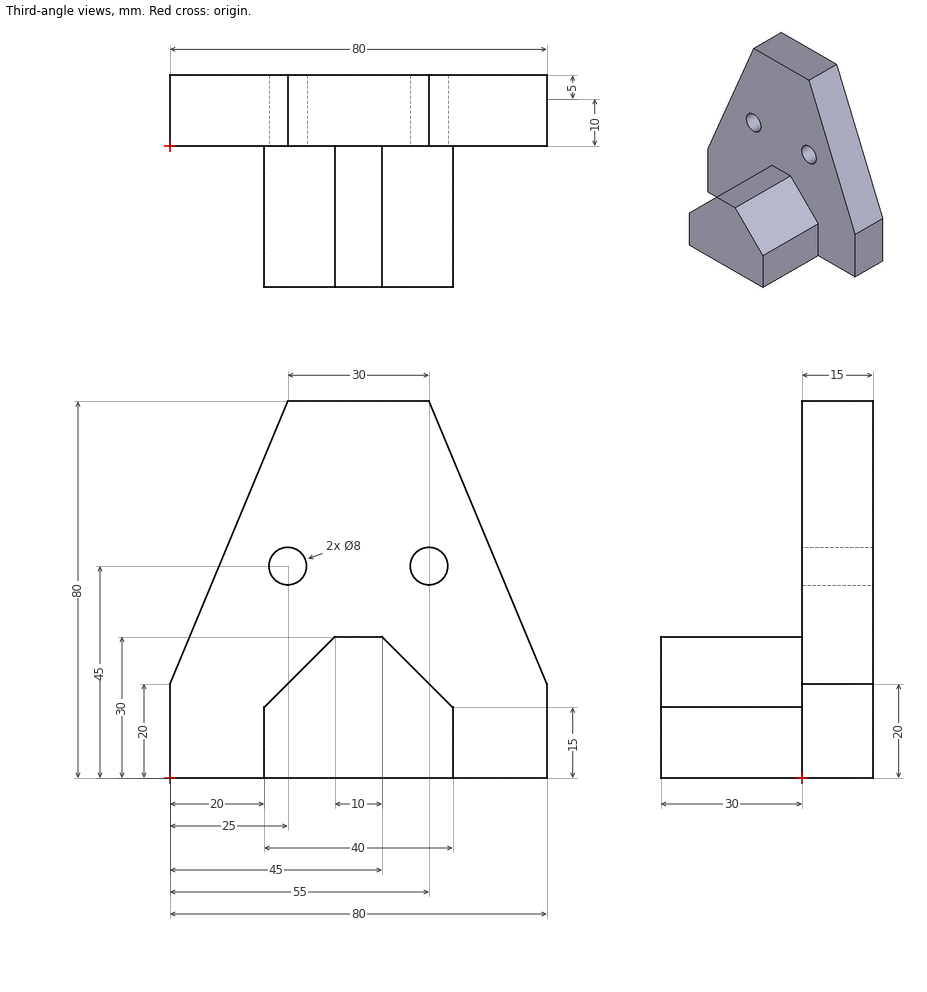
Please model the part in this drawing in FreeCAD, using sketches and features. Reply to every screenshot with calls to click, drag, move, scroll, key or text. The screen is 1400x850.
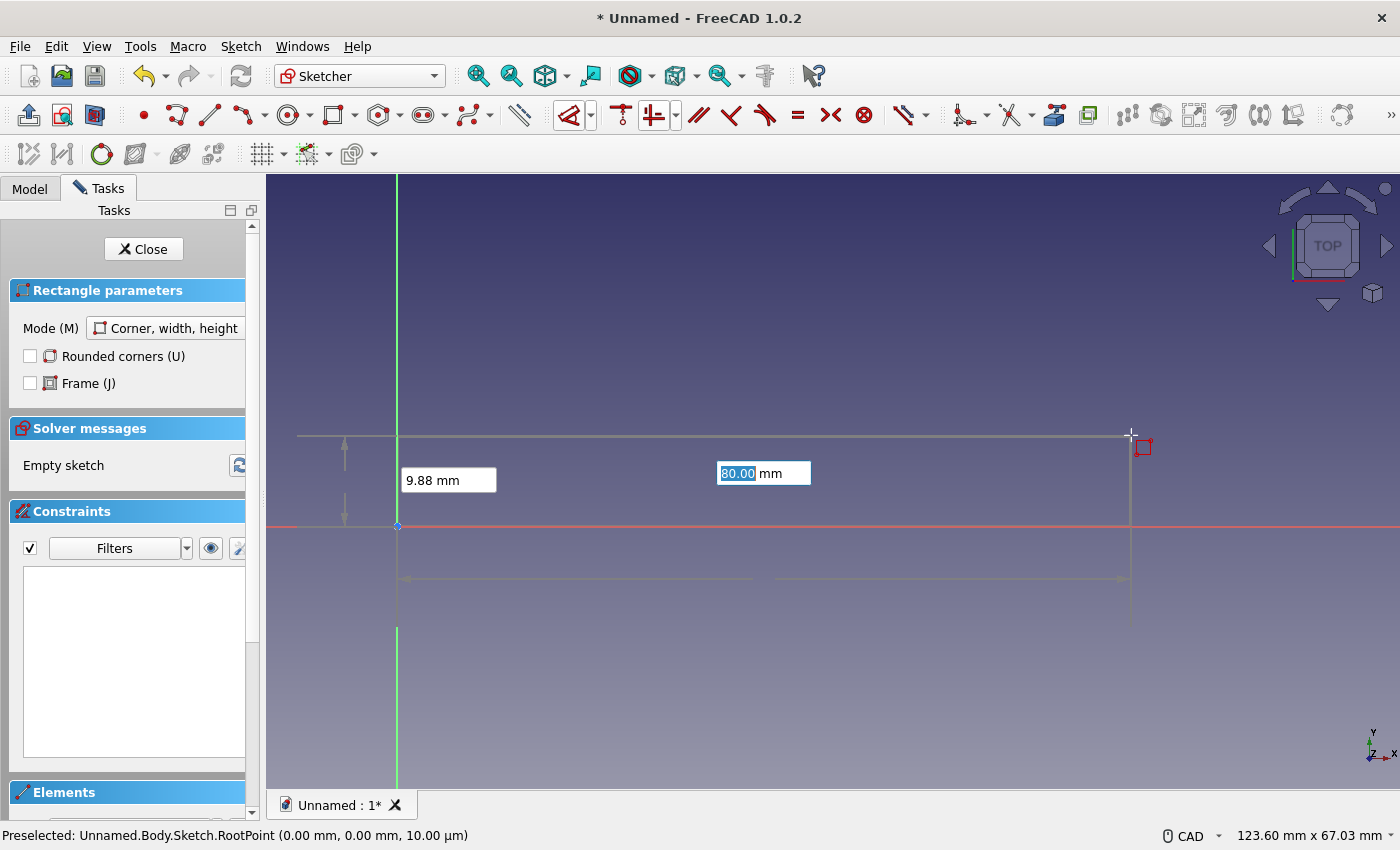
text(80)
key(Tab)
text(10)
key(Return)
key(Escape)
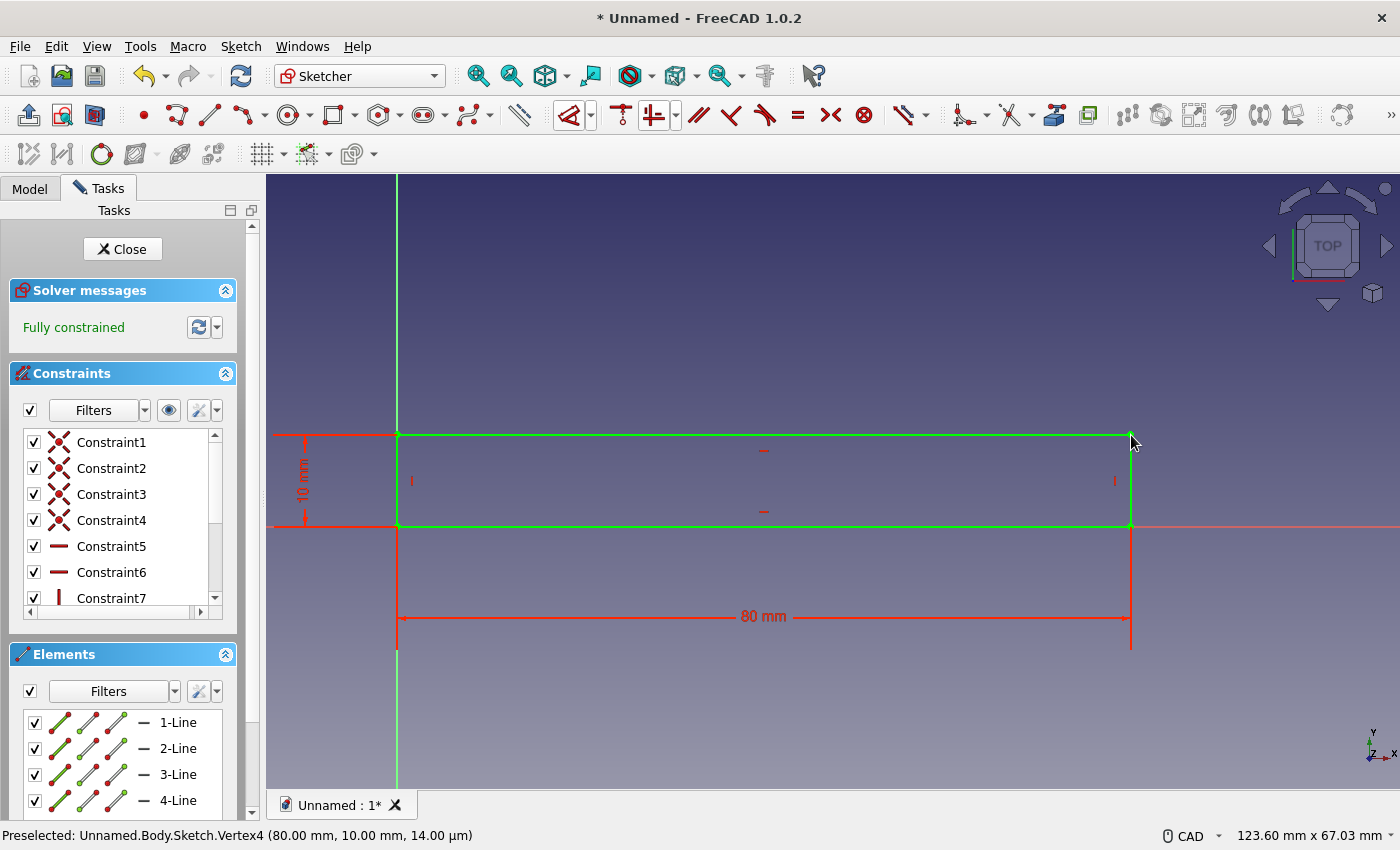
click(123, 249)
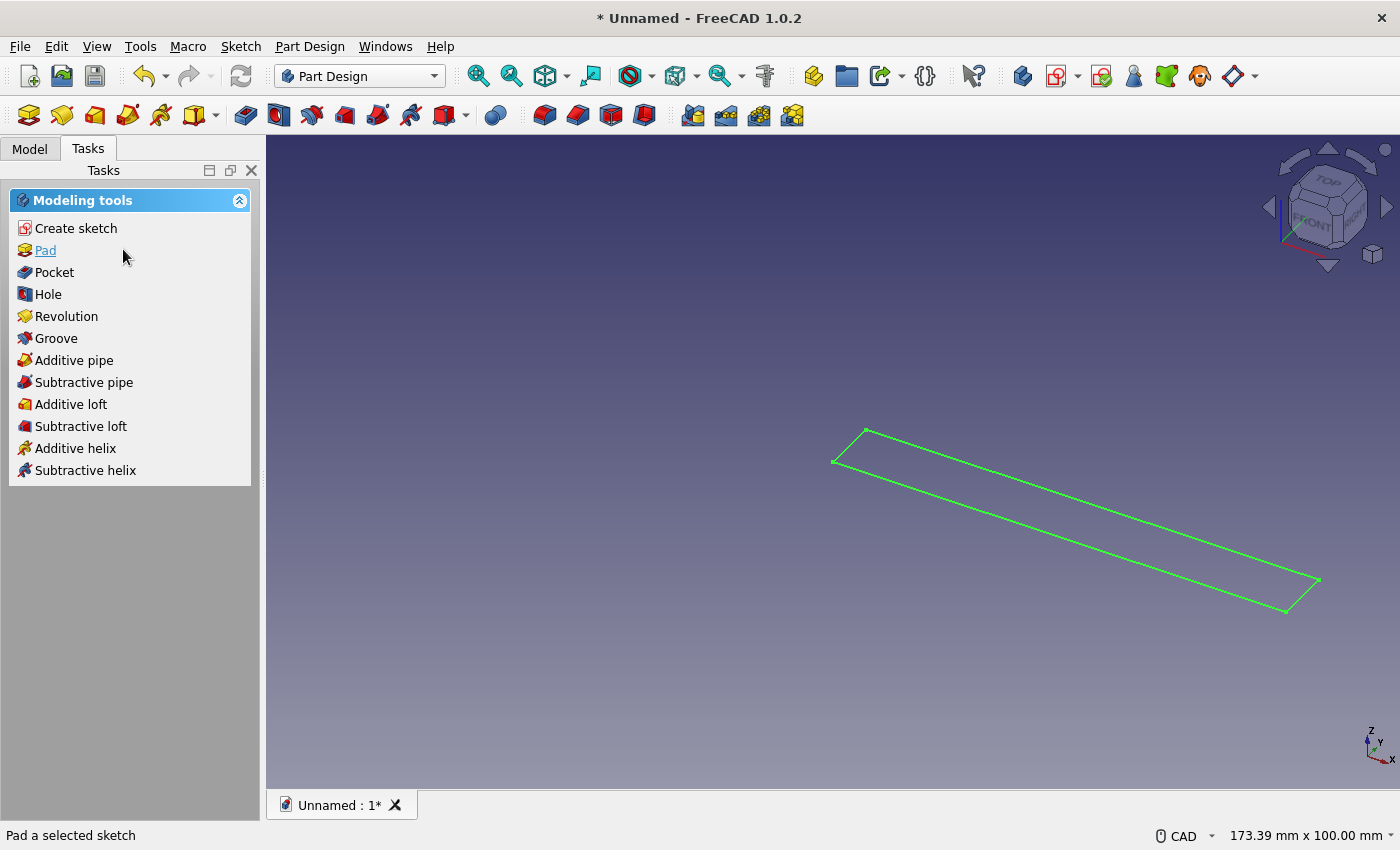
click(29, 116)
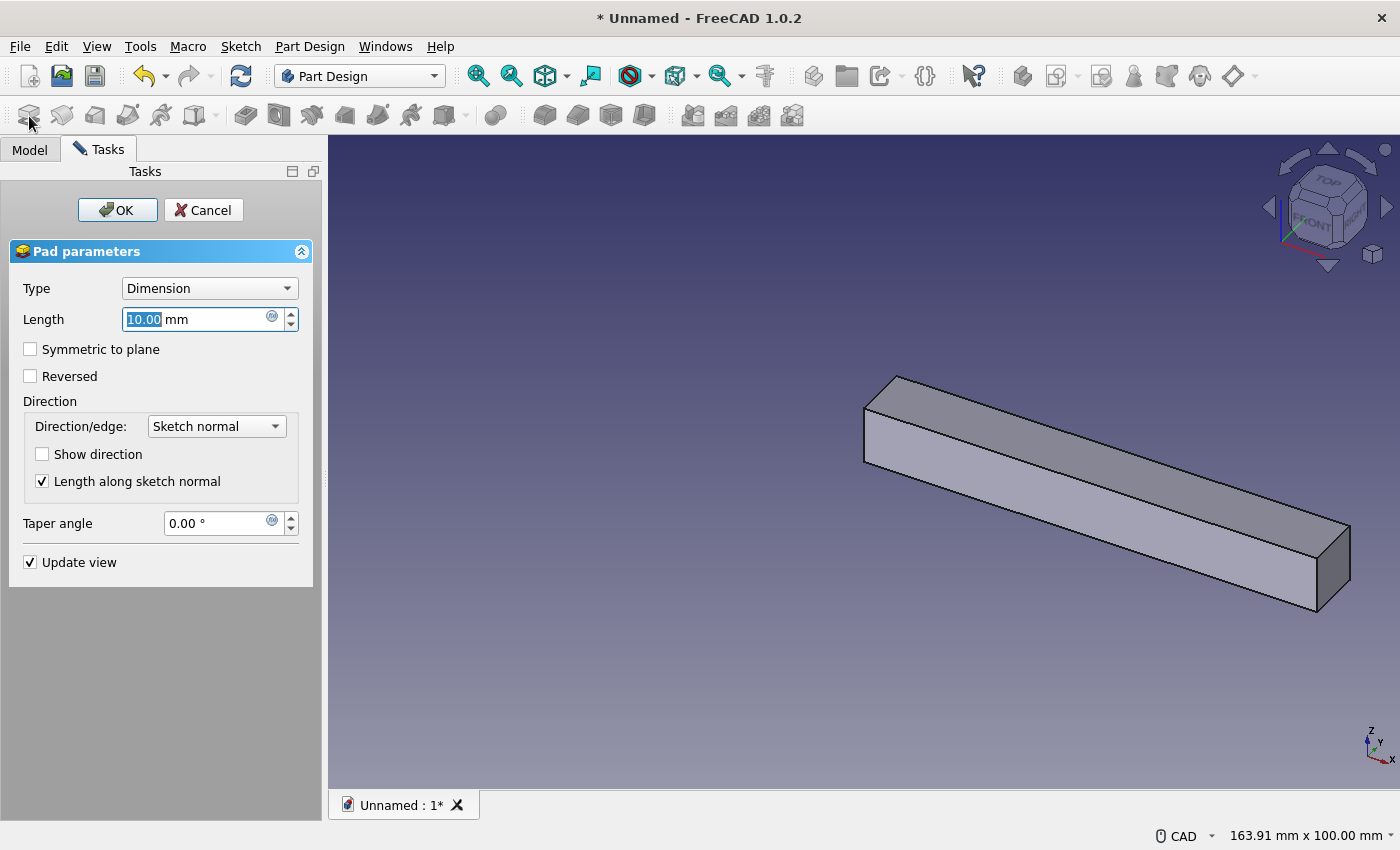
text(20)
key(Tab)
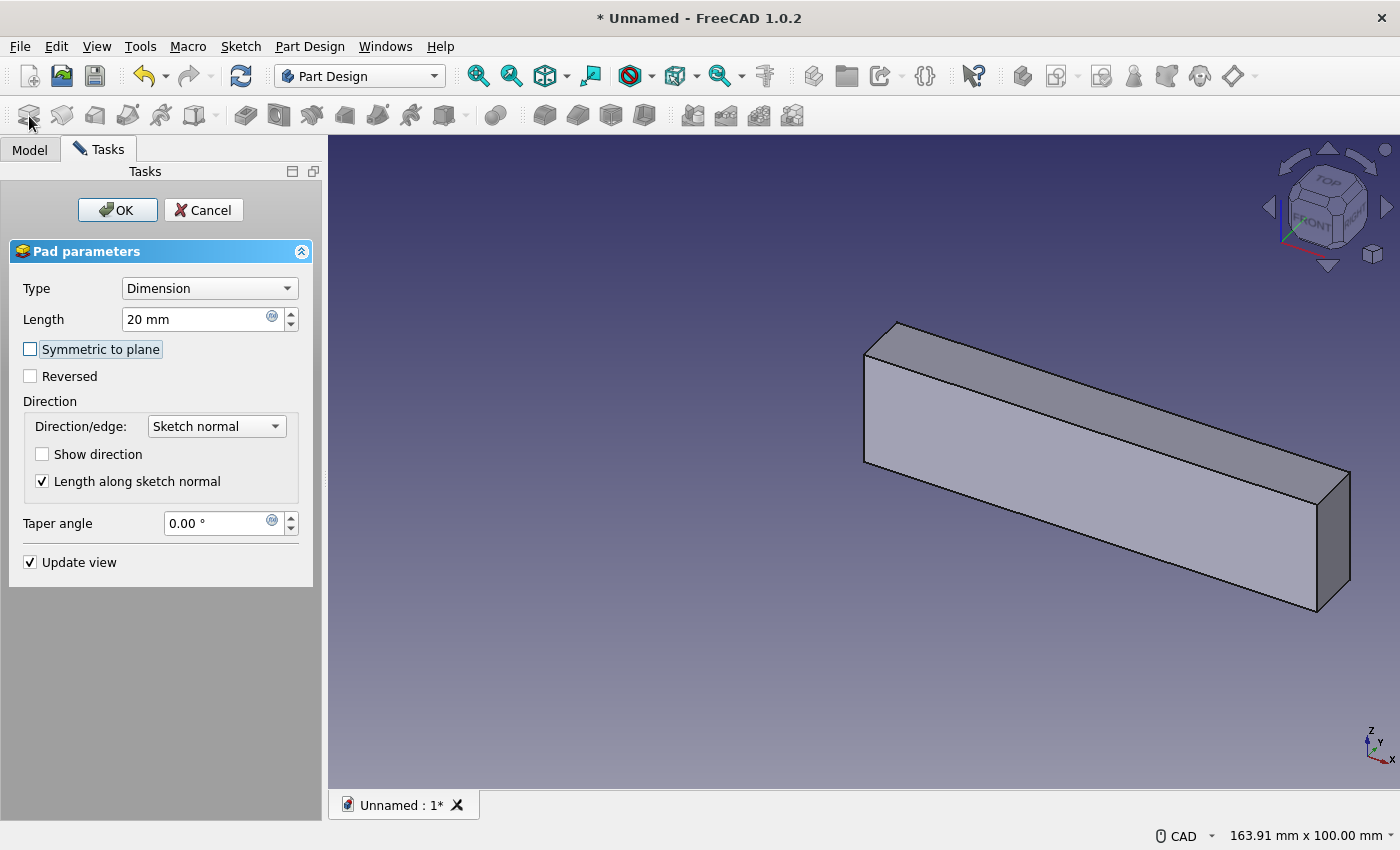
click(118, 210)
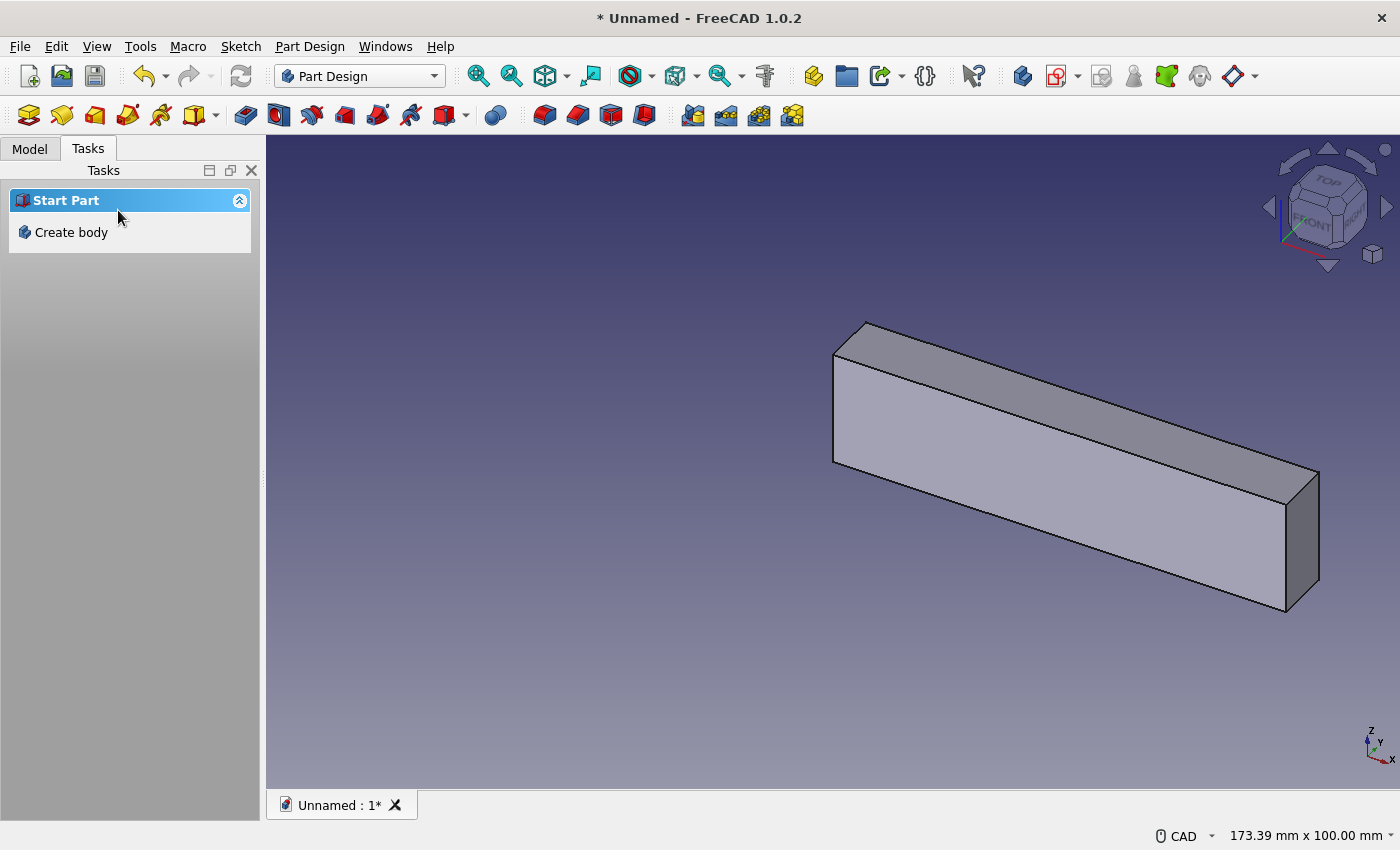
click(479, 76)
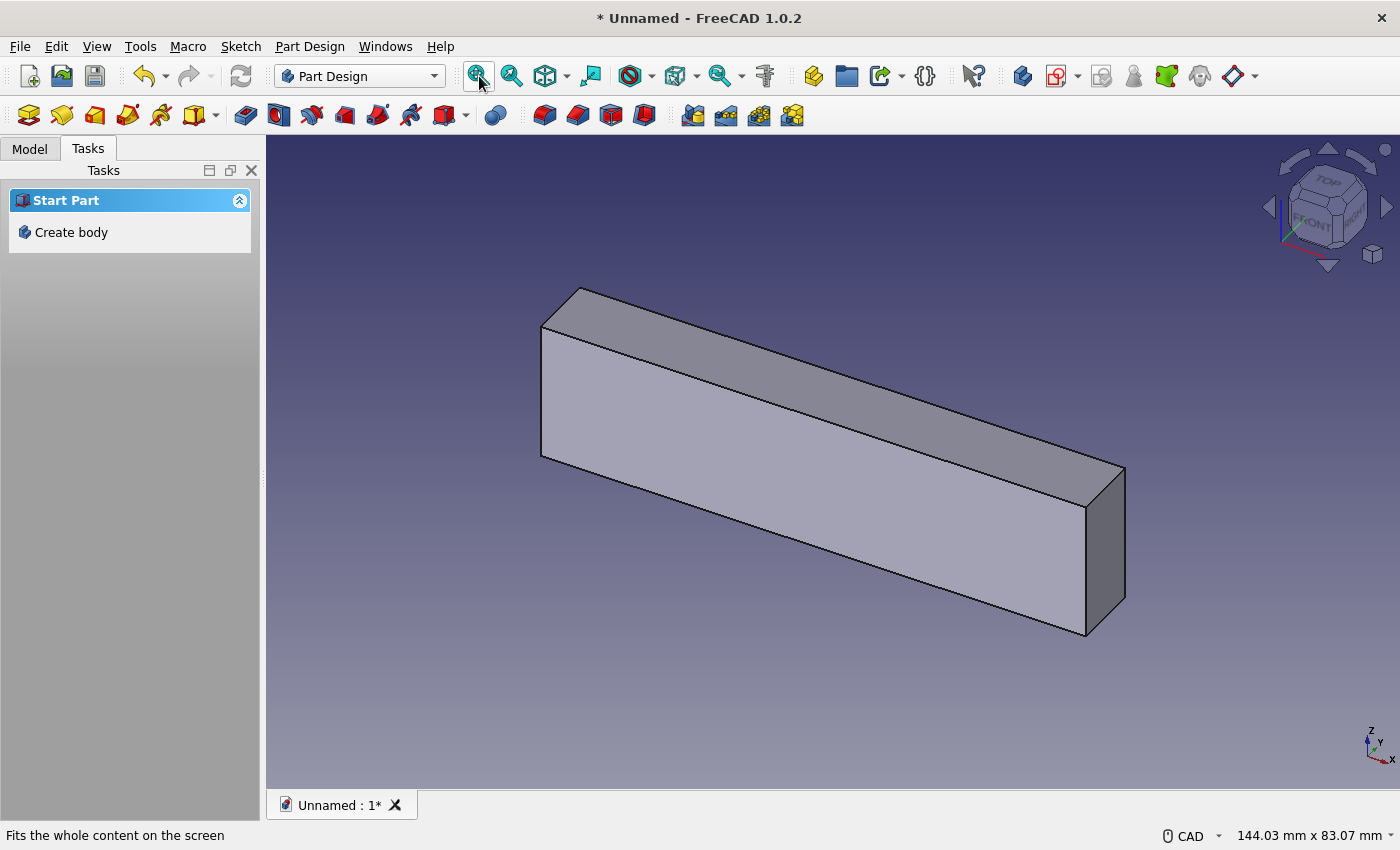
click(1056, 76)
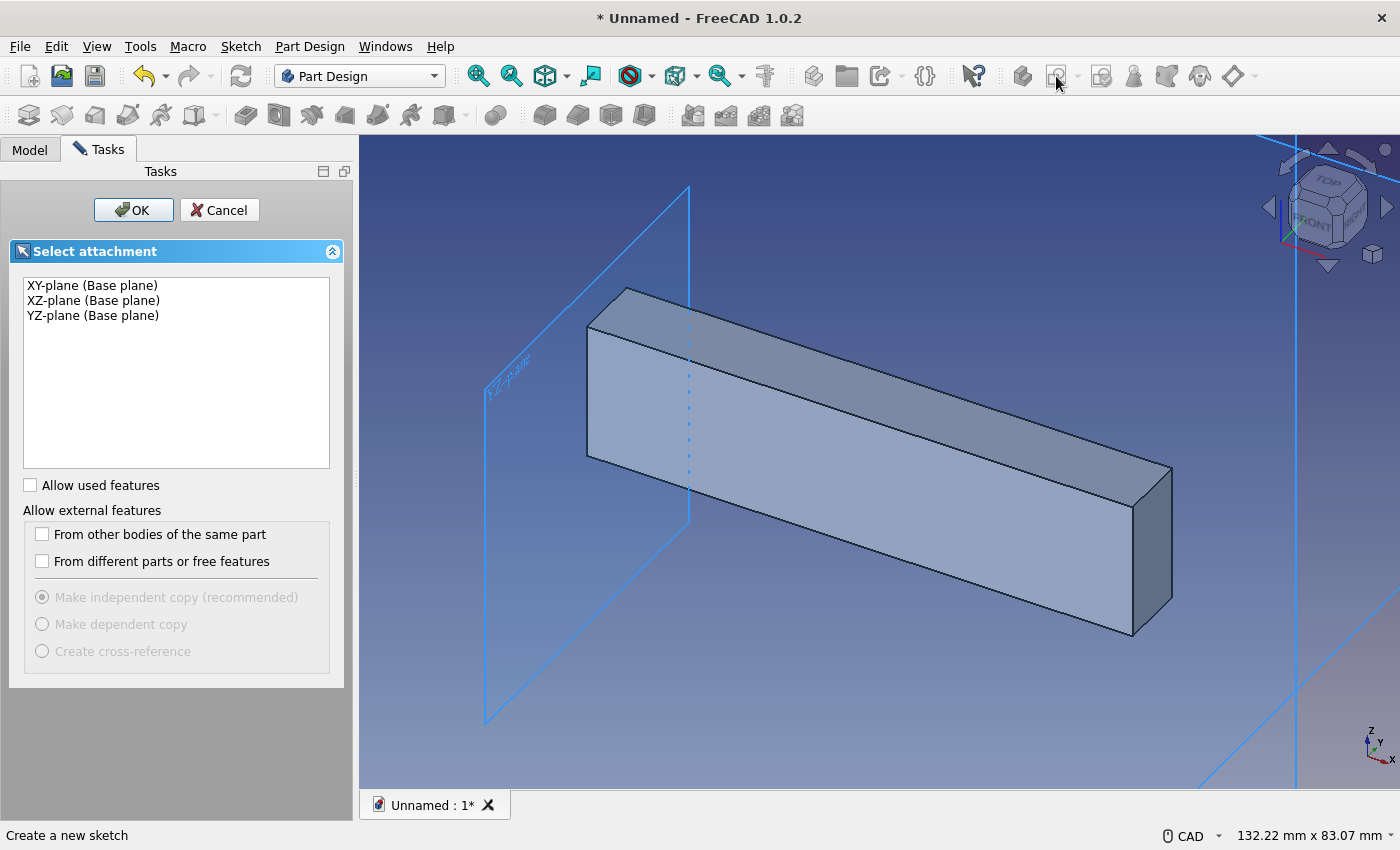
click(84, 300)